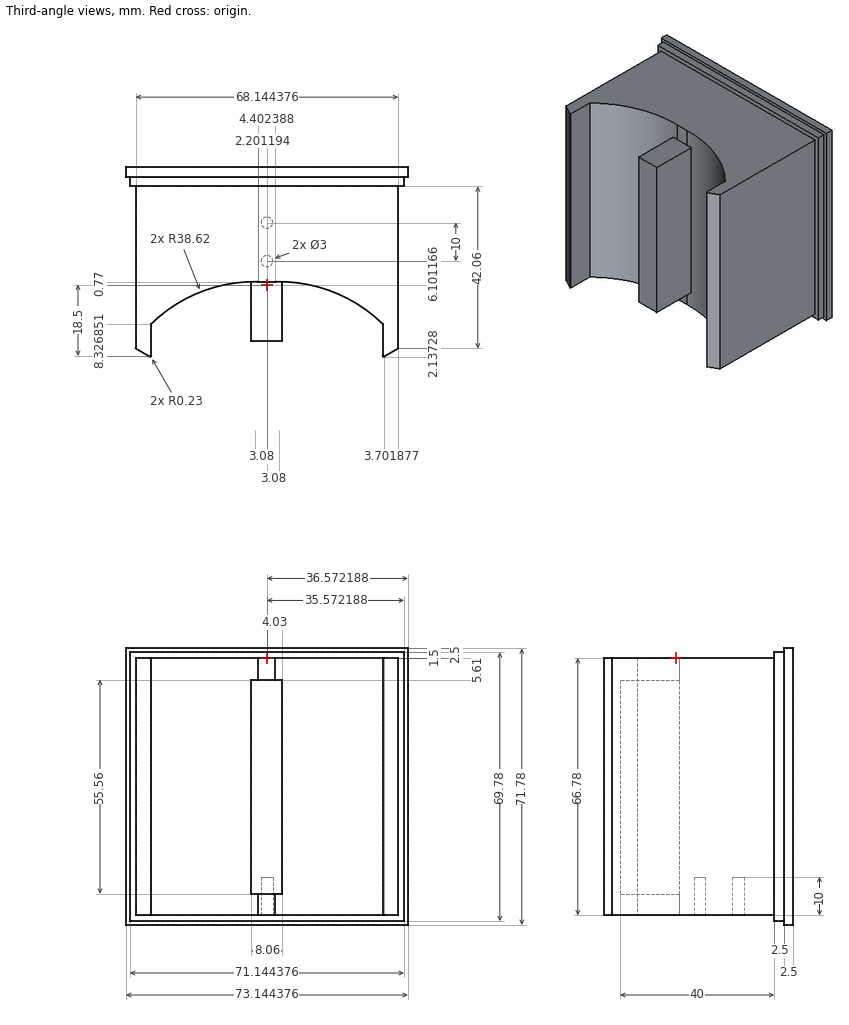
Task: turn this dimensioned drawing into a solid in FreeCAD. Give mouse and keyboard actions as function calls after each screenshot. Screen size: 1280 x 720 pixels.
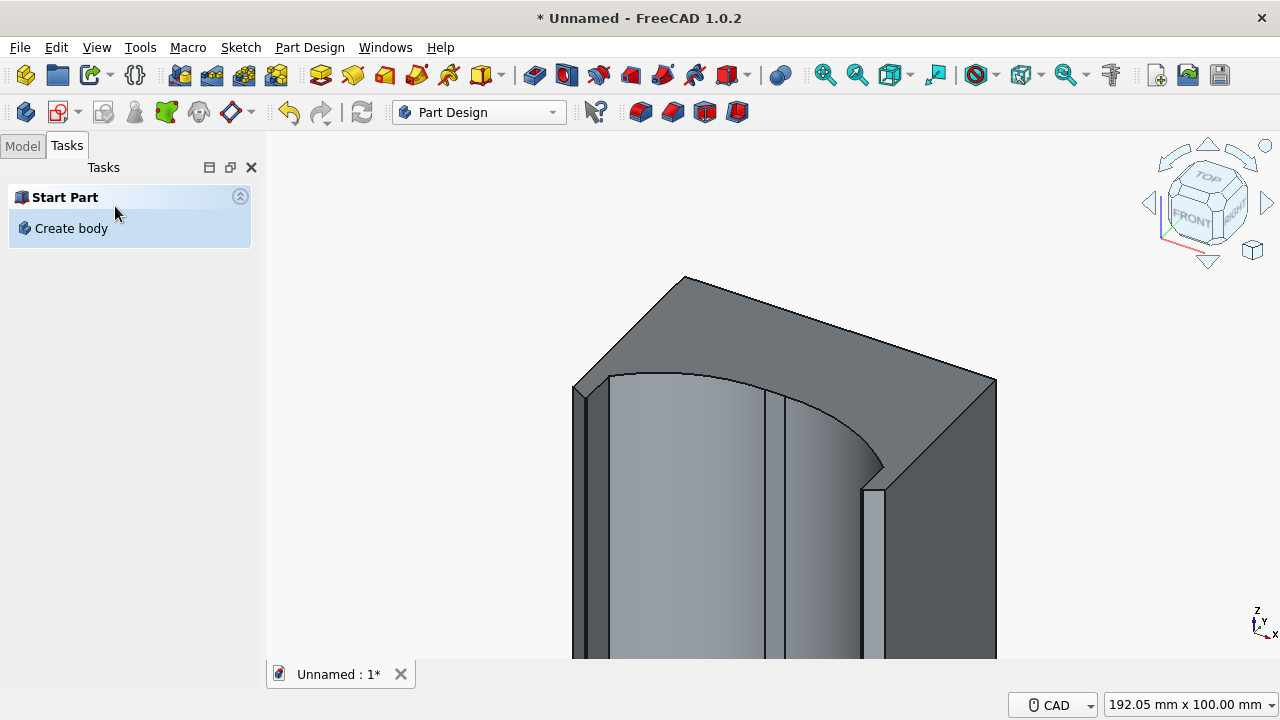
click(826, 76)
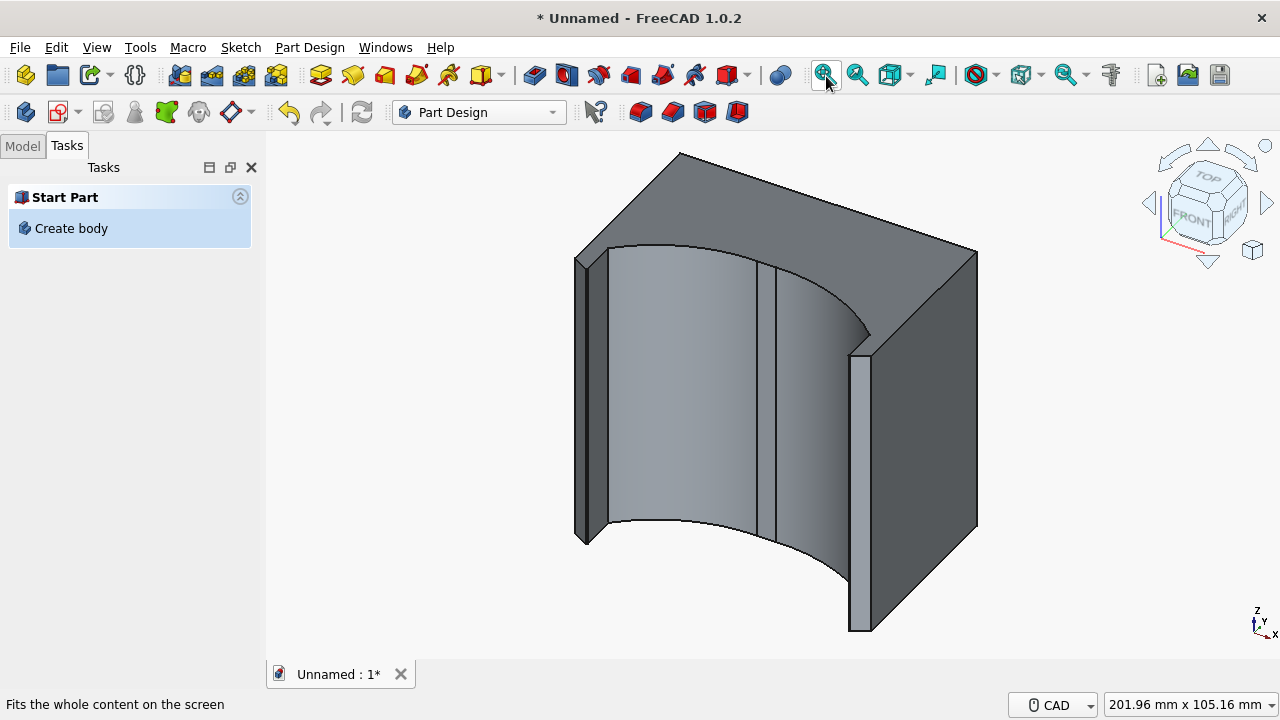
key(4)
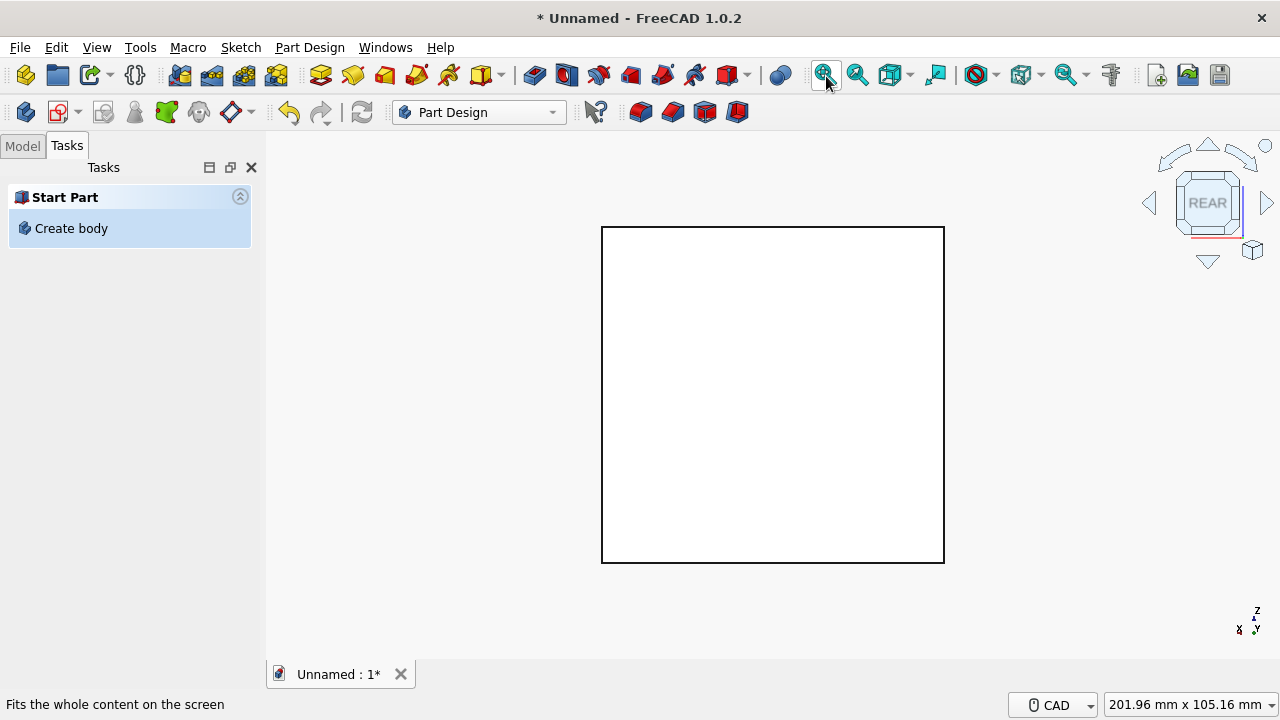
click(773, 394)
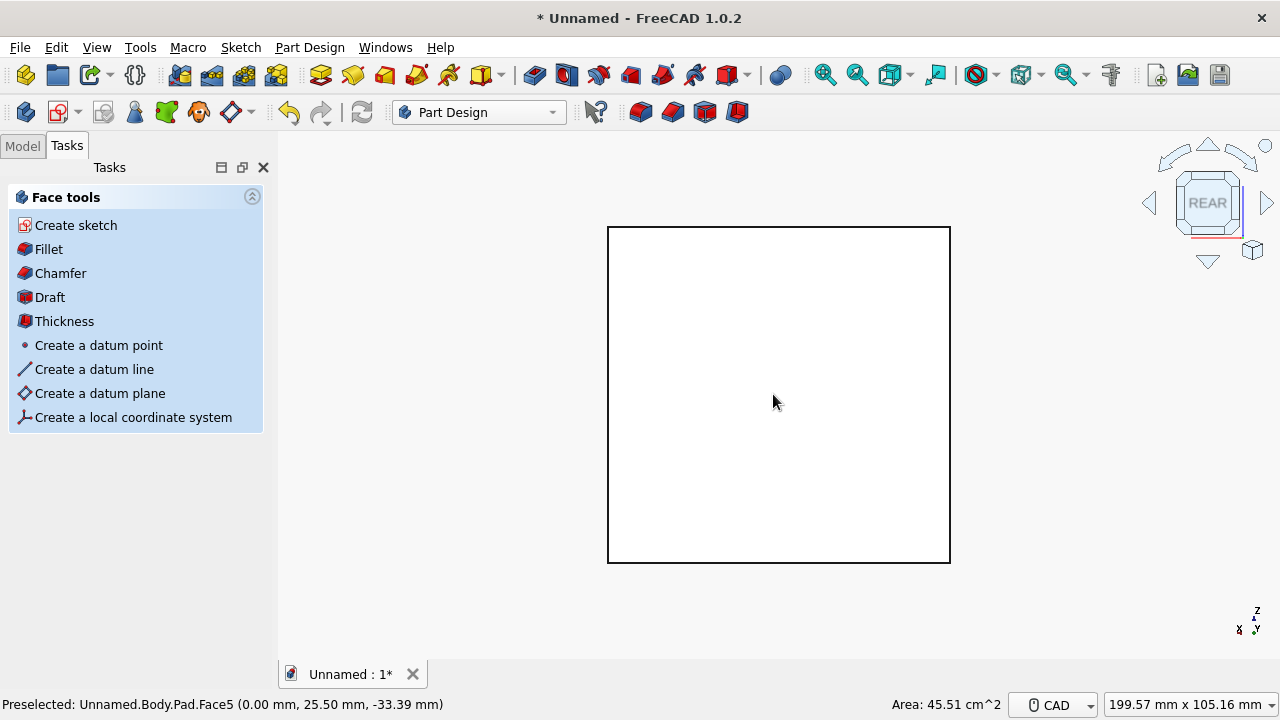
click(58, 112)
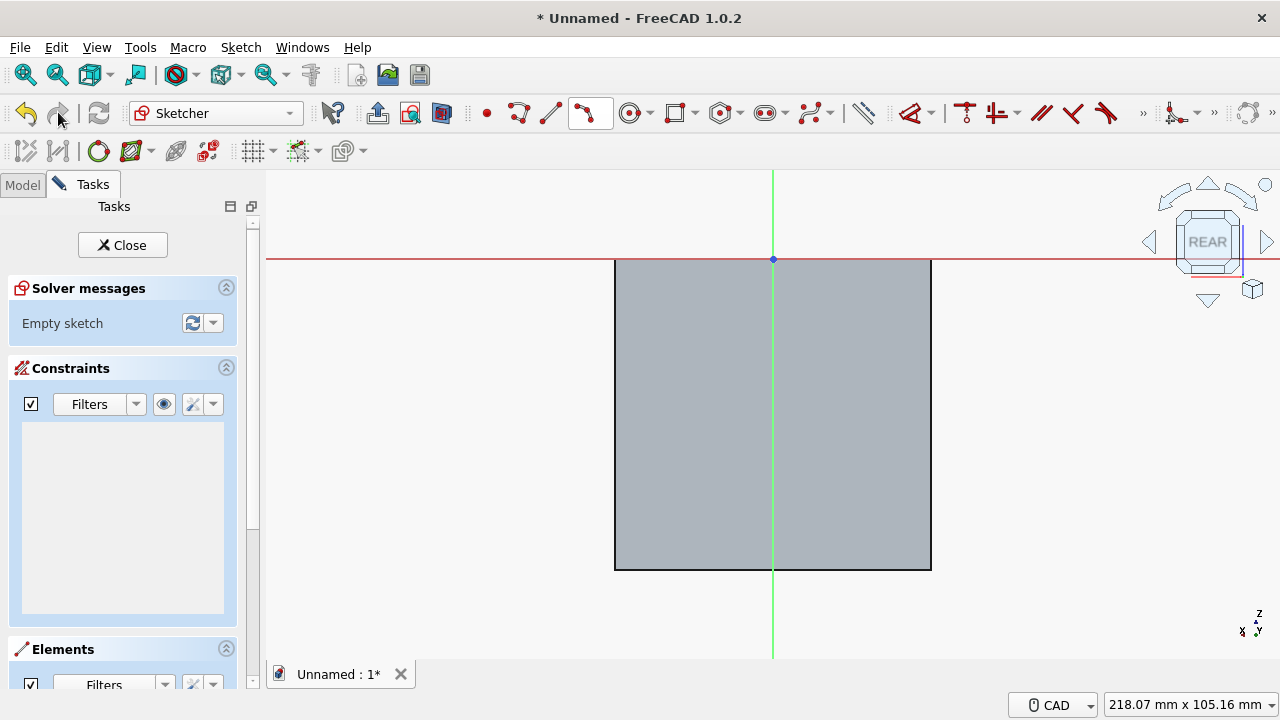
click(676, 114)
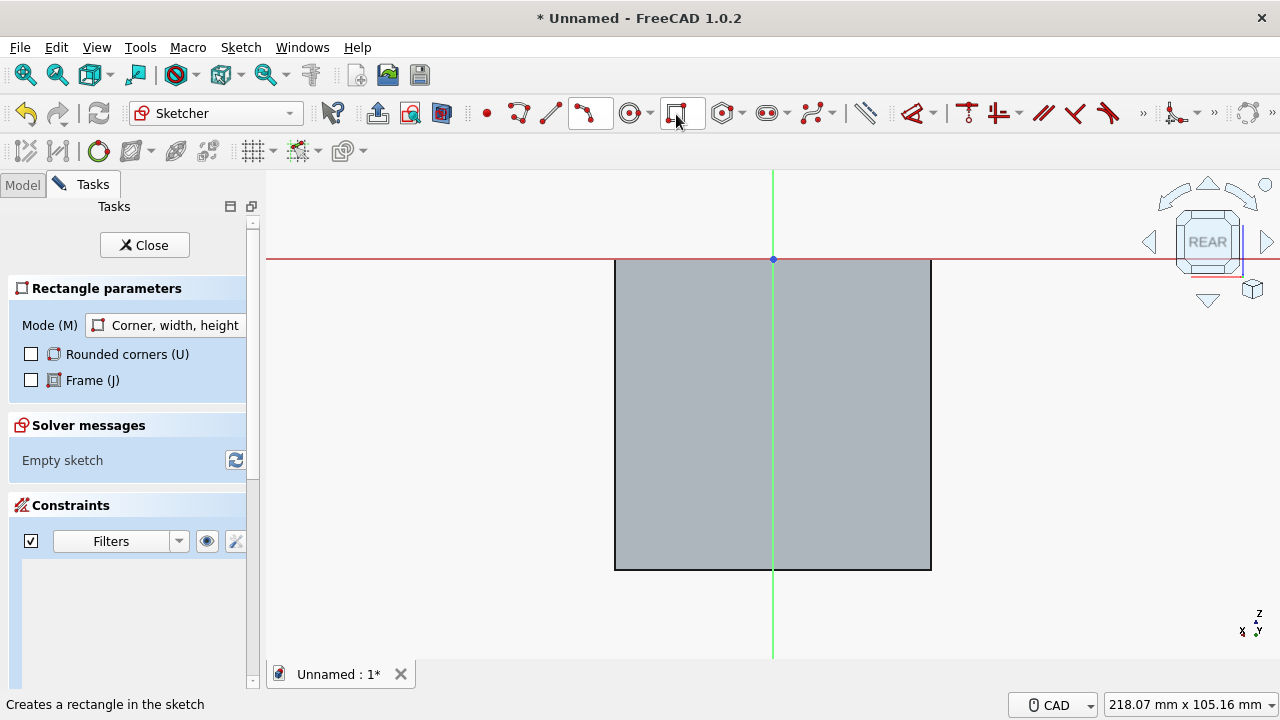
click(754, 285)
move(792, 544)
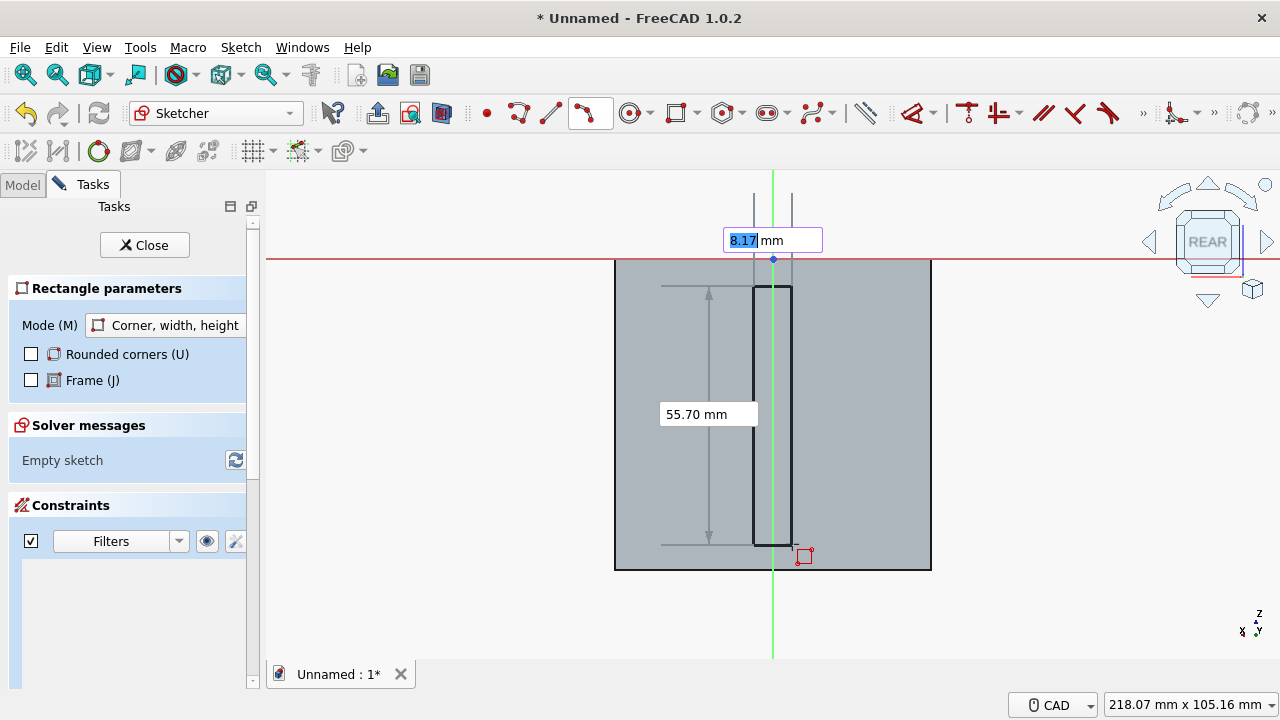
text(8.06)
key(Tab)
text(55.56)
key(Return)
key(Escape)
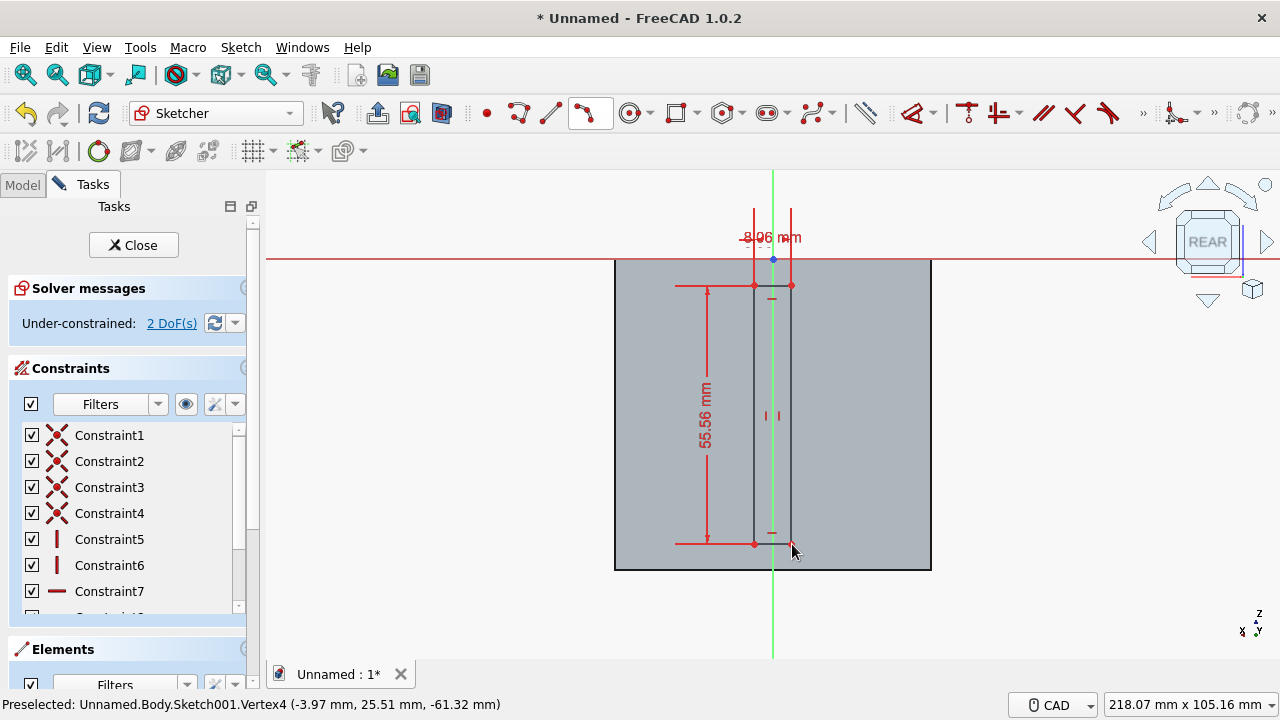
click(912, 114)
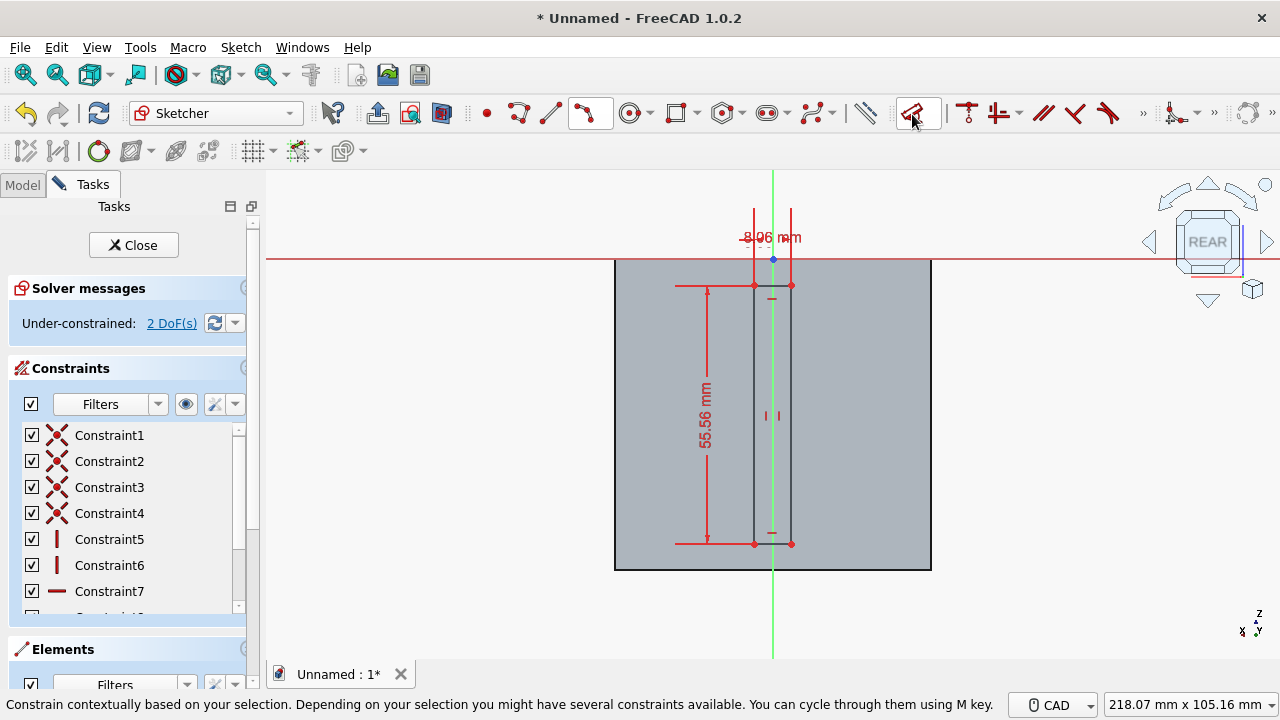
scroll(754, 286, up, 4)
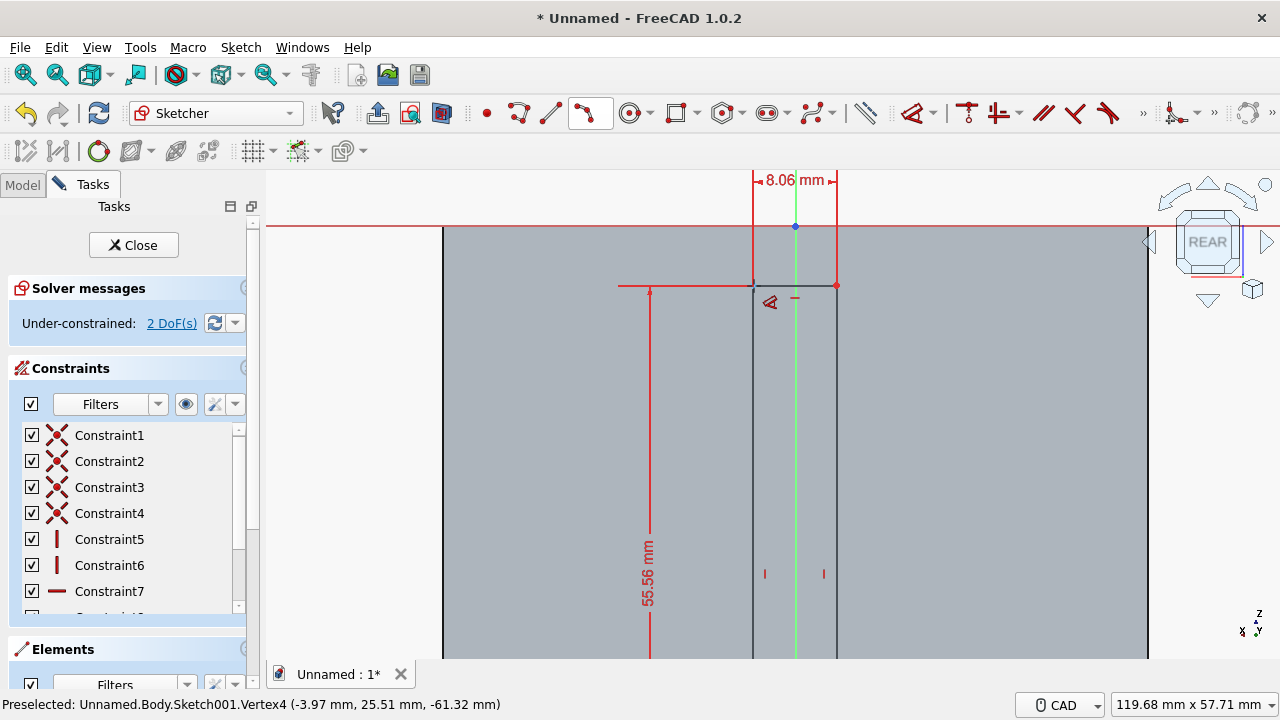
click(753, 286)
click(775, 320)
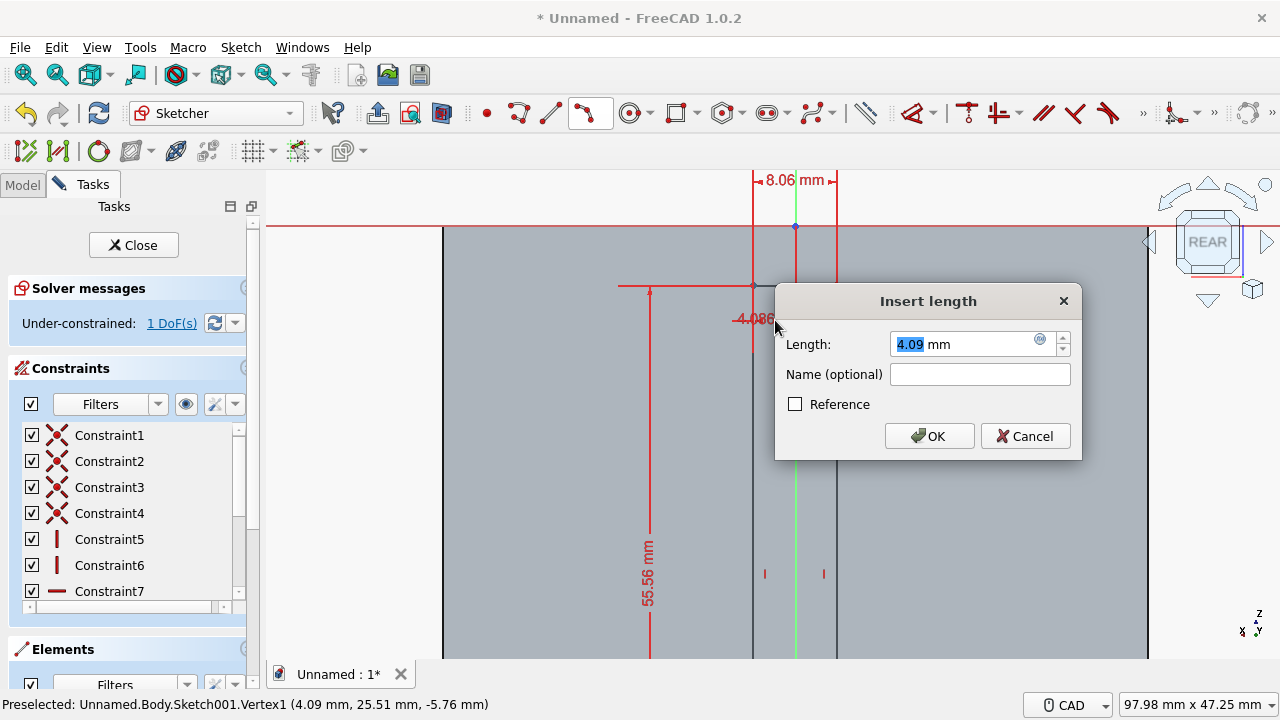
text(4.03)
key(Return)